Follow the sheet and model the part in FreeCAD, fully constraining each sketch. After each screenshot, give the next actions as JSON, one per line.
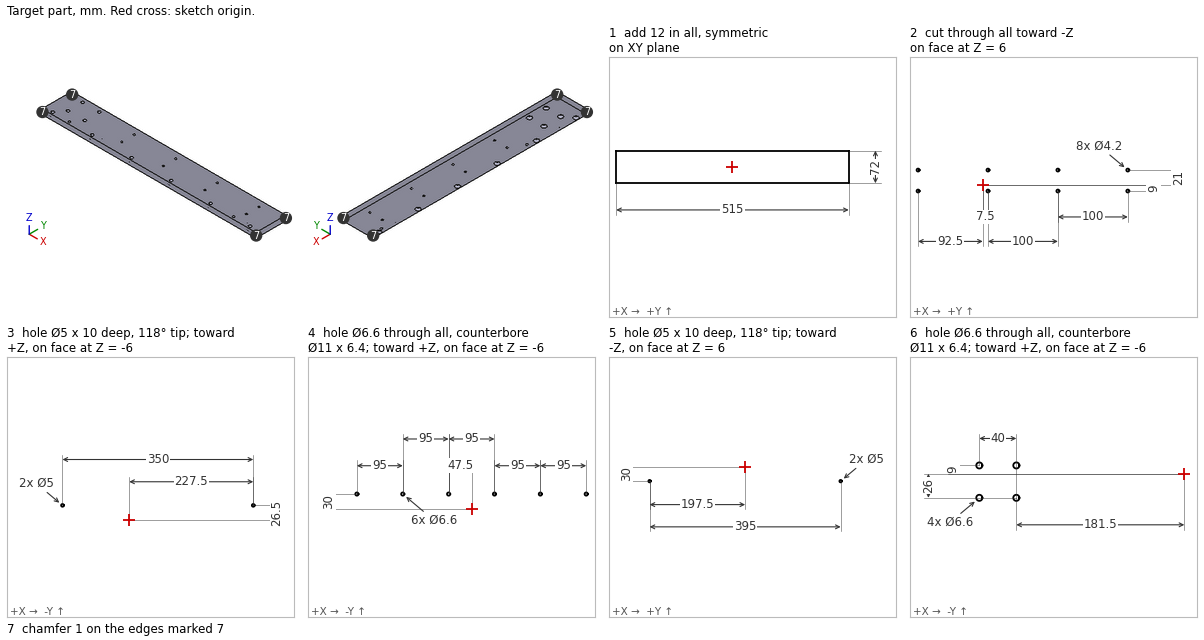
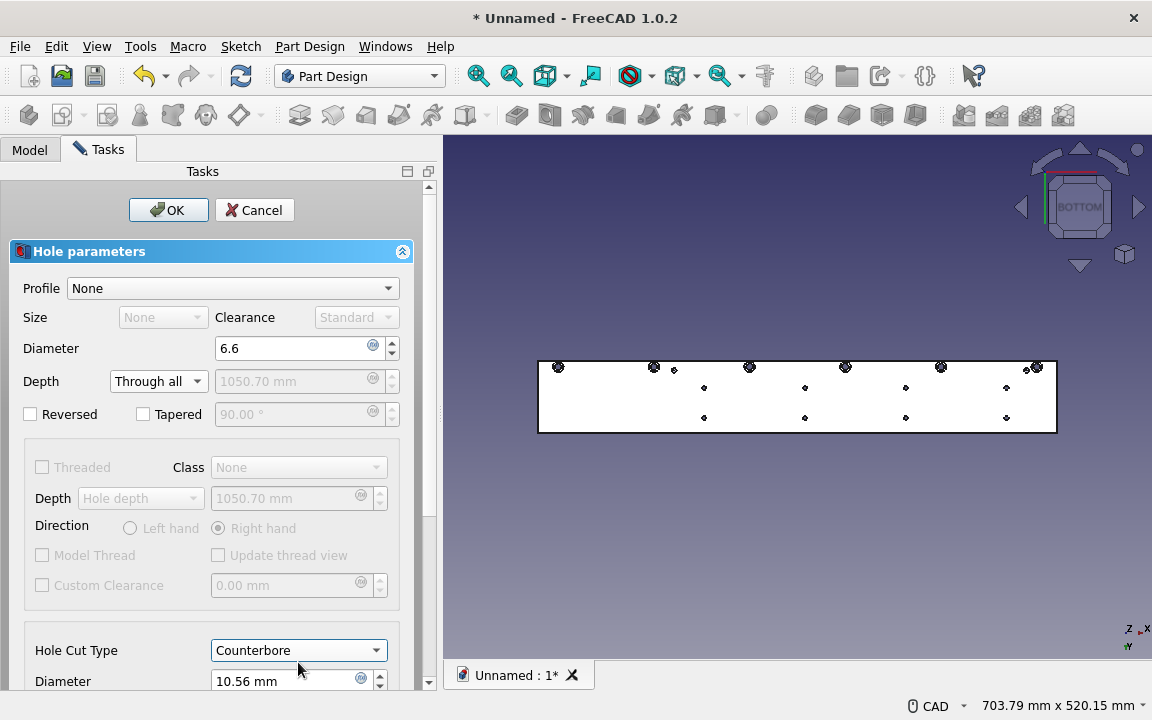
{"action": "scroll", "coordinate": [429, 436], "scroll_direction": "down", "scroll_amount": 2}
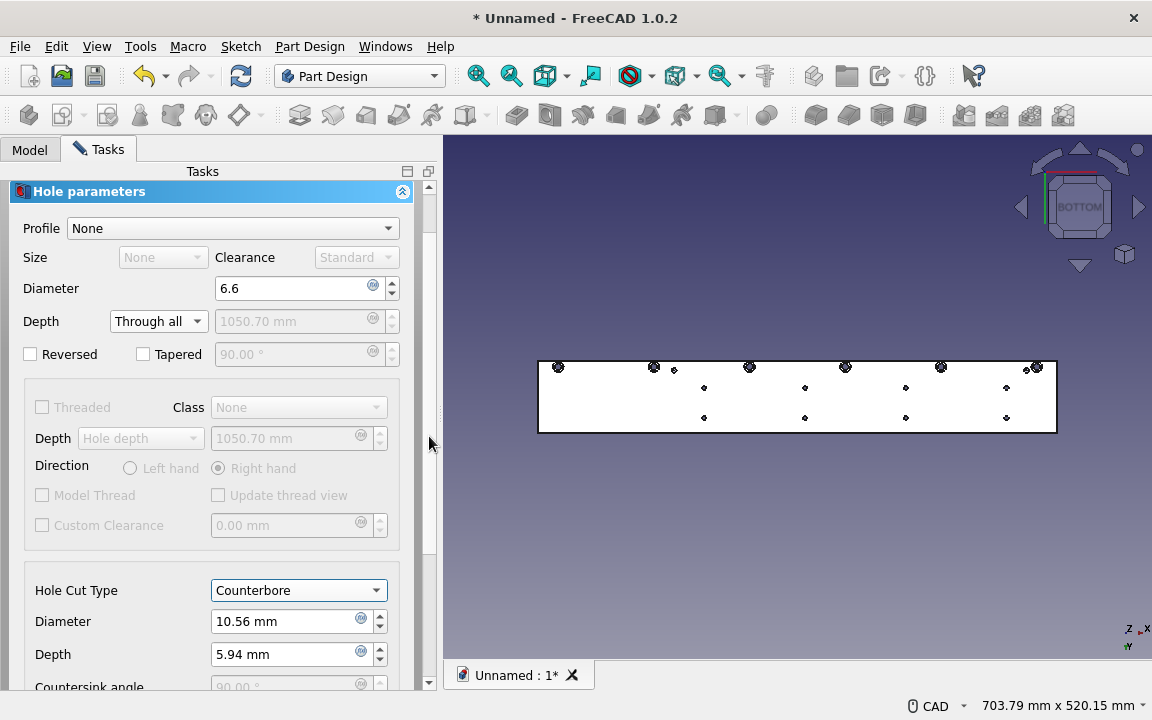
{"action": "triple_click", "coordinate": [292, 562]}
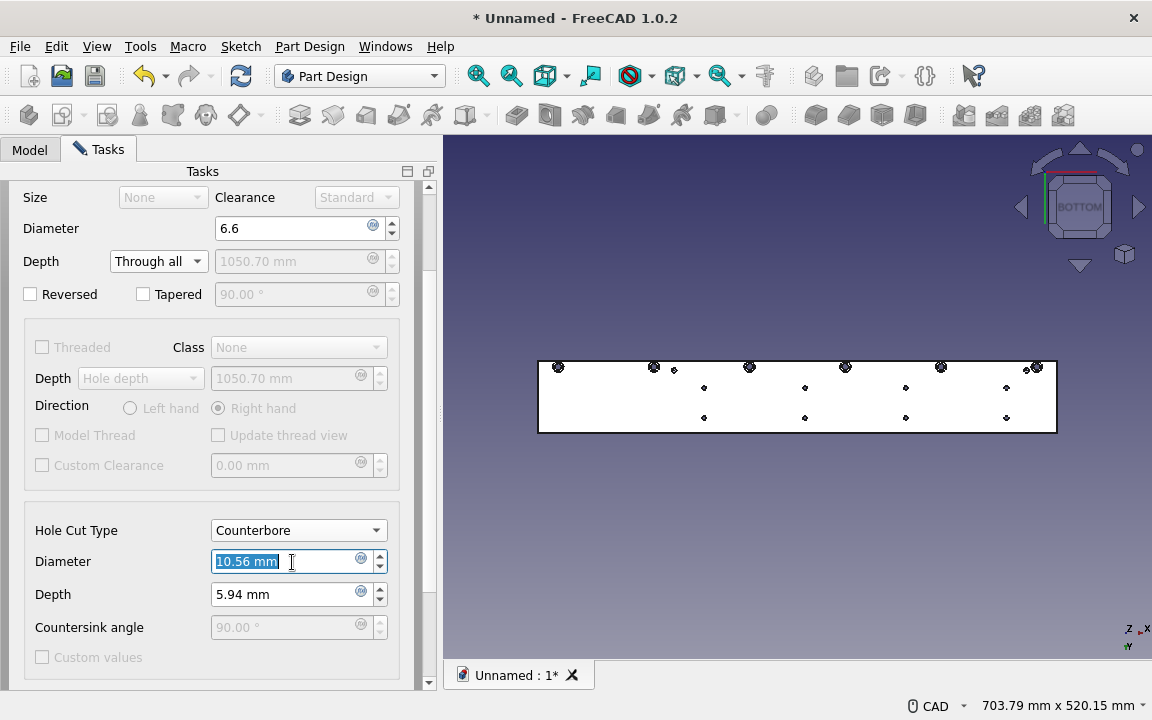
{"action": "type", "text": "11"}
{"action": "key", "text": "Tab"}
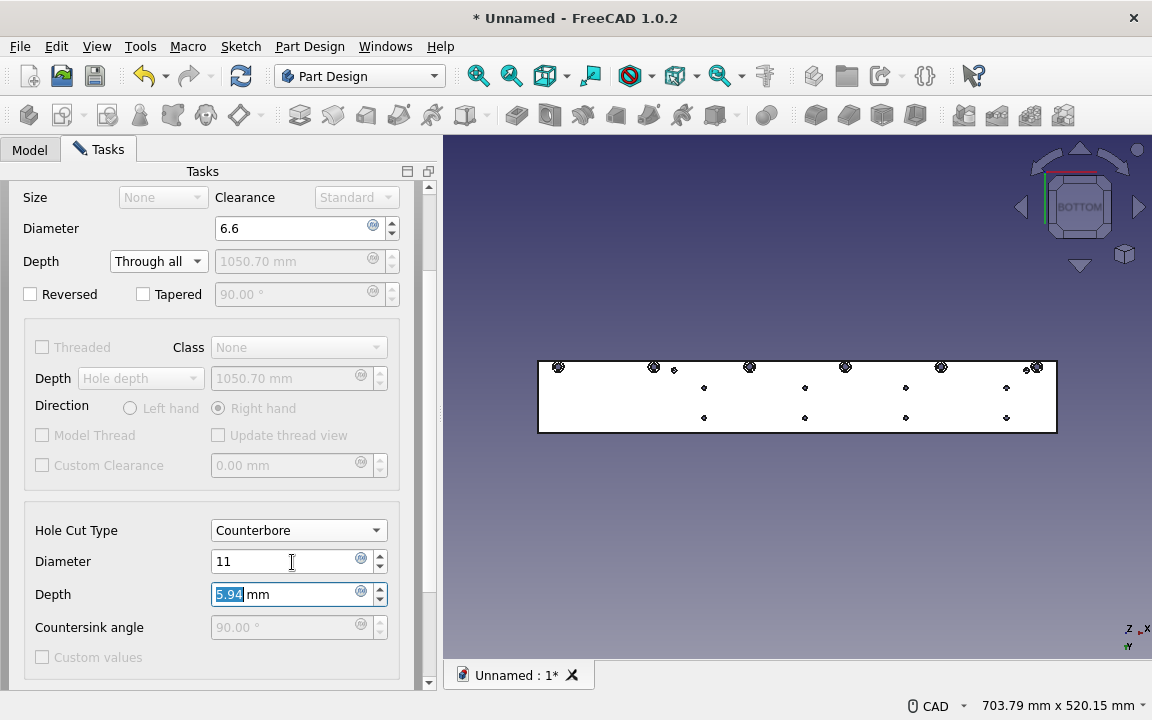
{"action": "type", "text": "6.4"}
{"action": "key", "text": "Tab"}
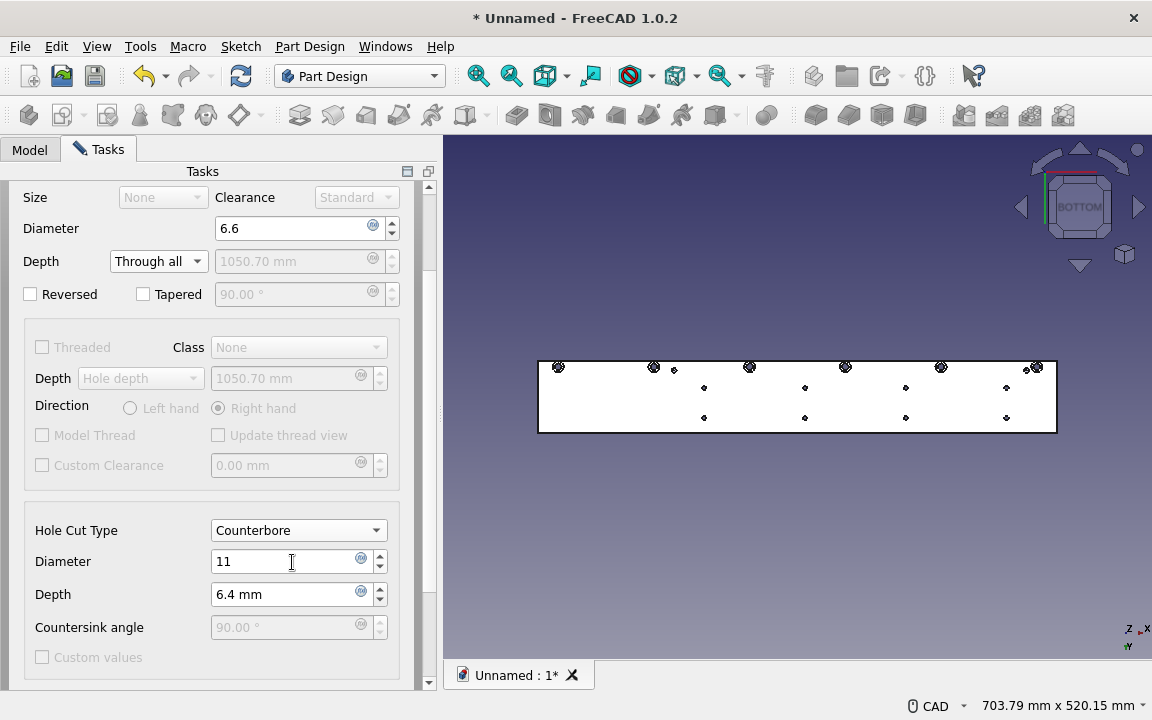
{"action": "scroll", "coordinate": [429, 436], "scroll_direction": "up", "scroll_amount": 3}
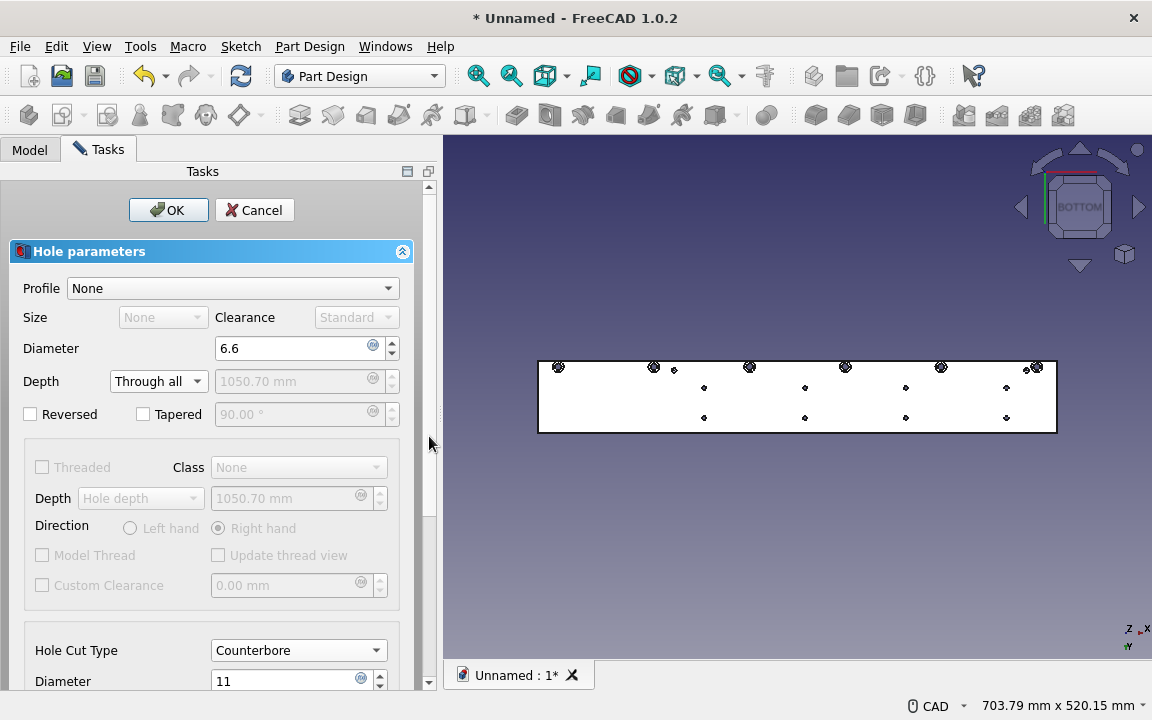
{"action": "left_click", "coordinate": [169, 210]}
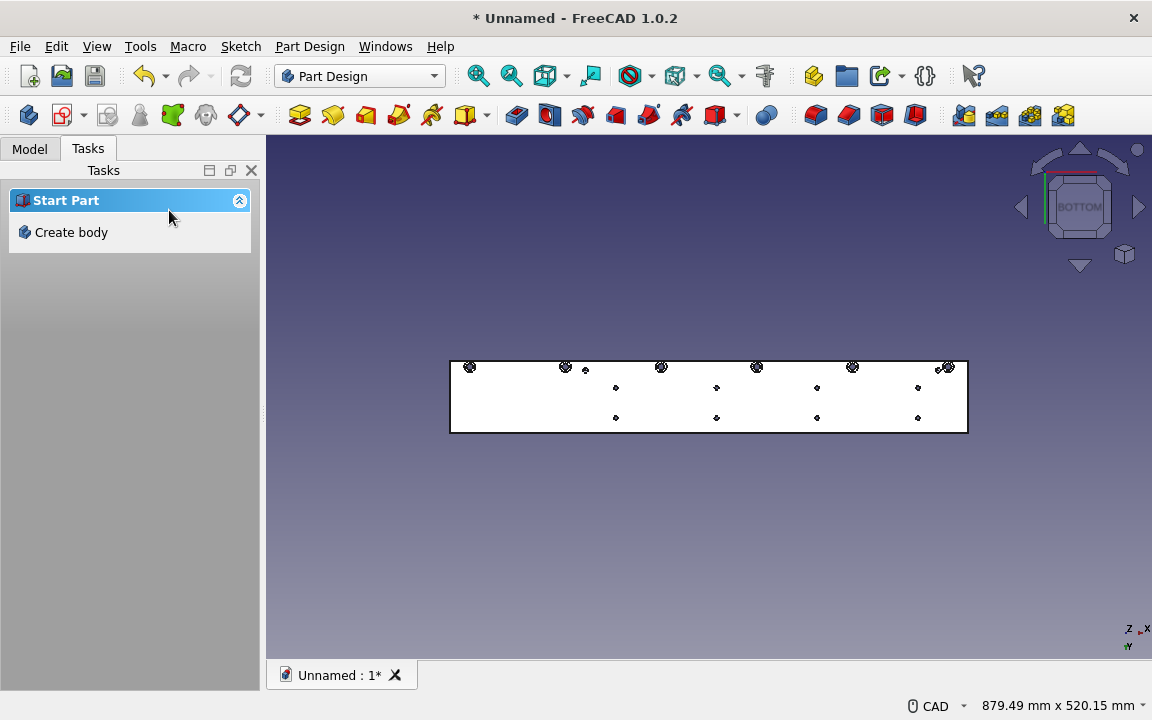
{"action": "key", "text": "0"}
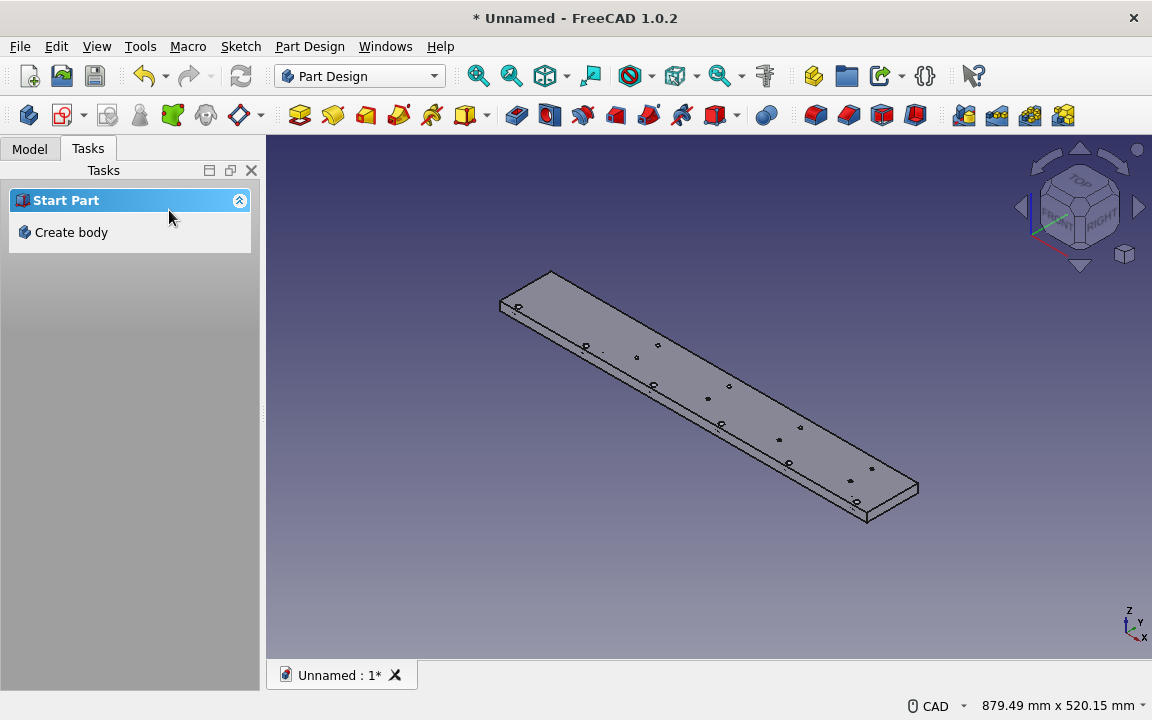
{"action": "left_click", "coordinate": [761, 421]}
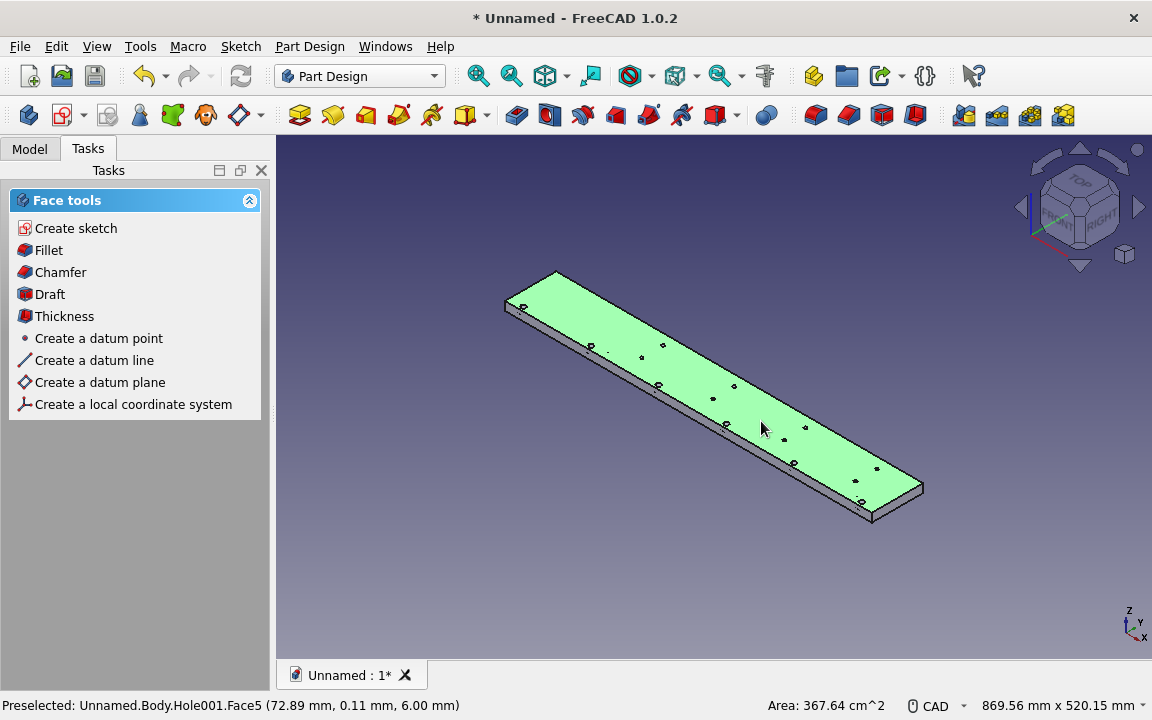
{"action": "left_click", "coordinate": [62, 116]}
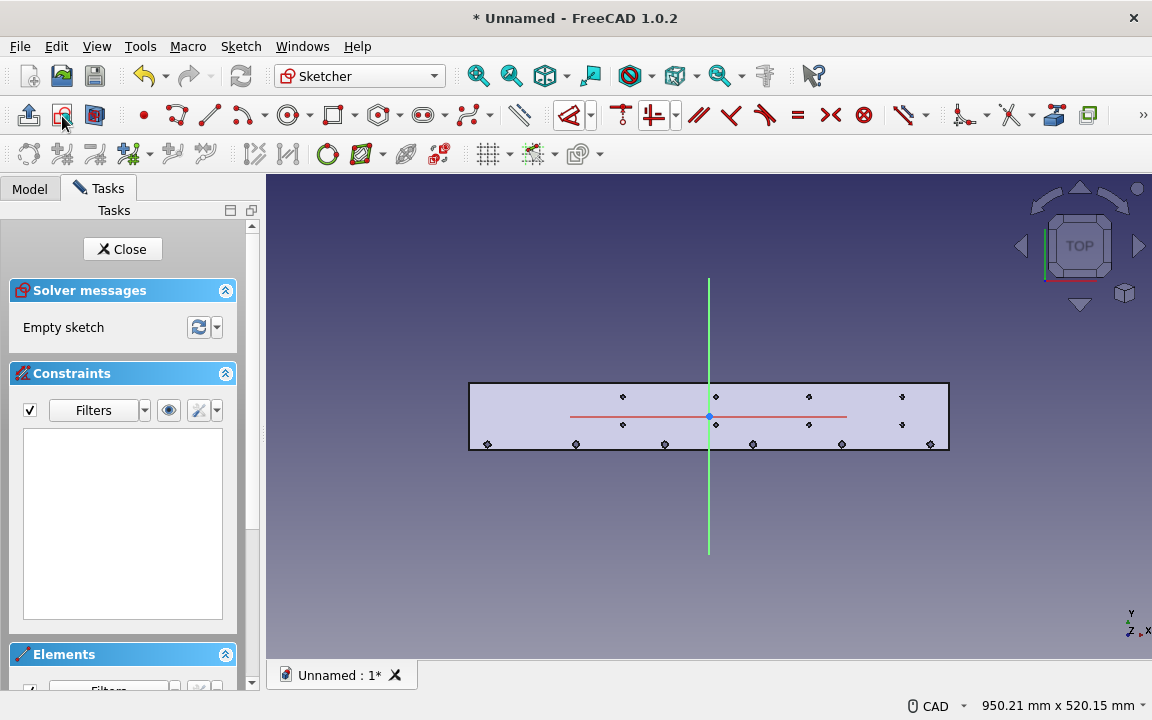
{"action": "left_click", "coordinate": [288, 116]}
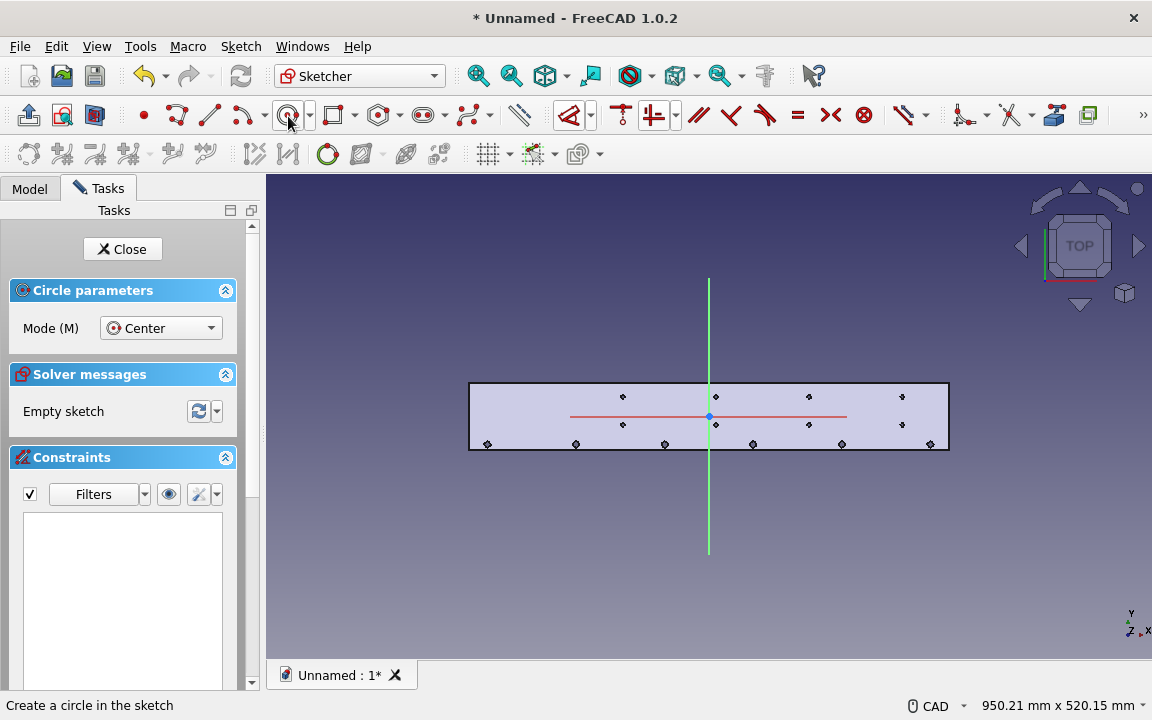
{"action": "scroll", "coordinate": [525, 444], "scroll_direction": "up", "scroll_amount": 12}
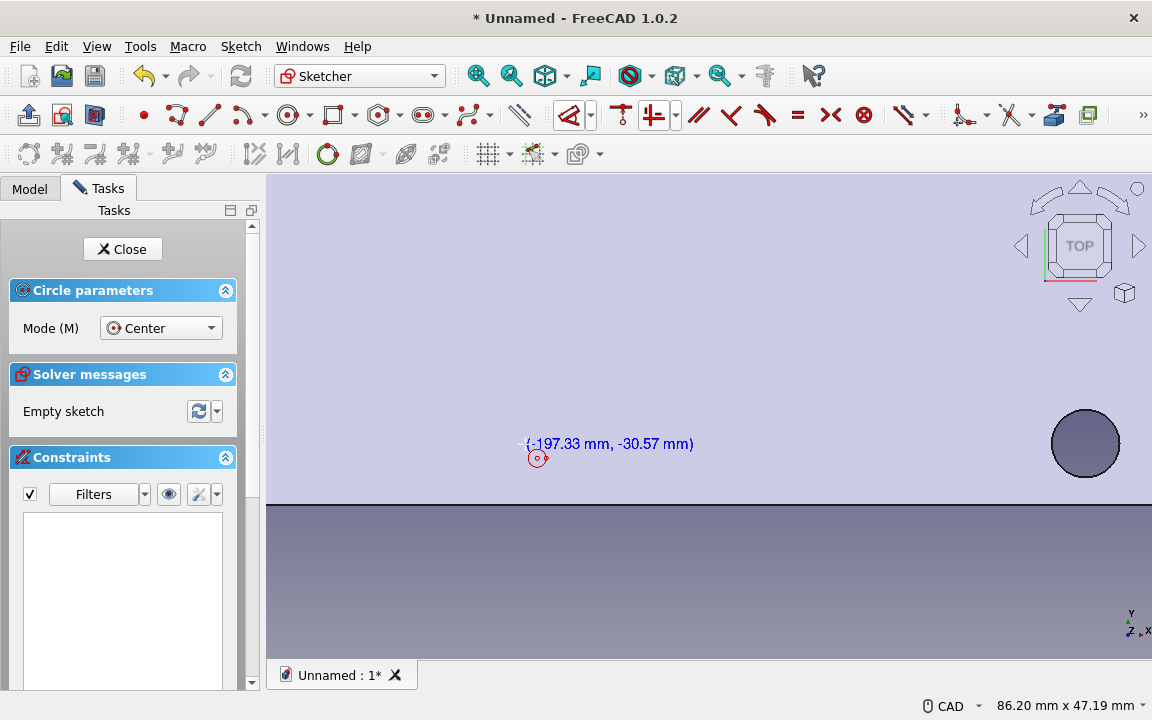
{"action": "scroll", "coordinate": [403, 431], "scroll_direction": "down", "scroll_amount": 11}